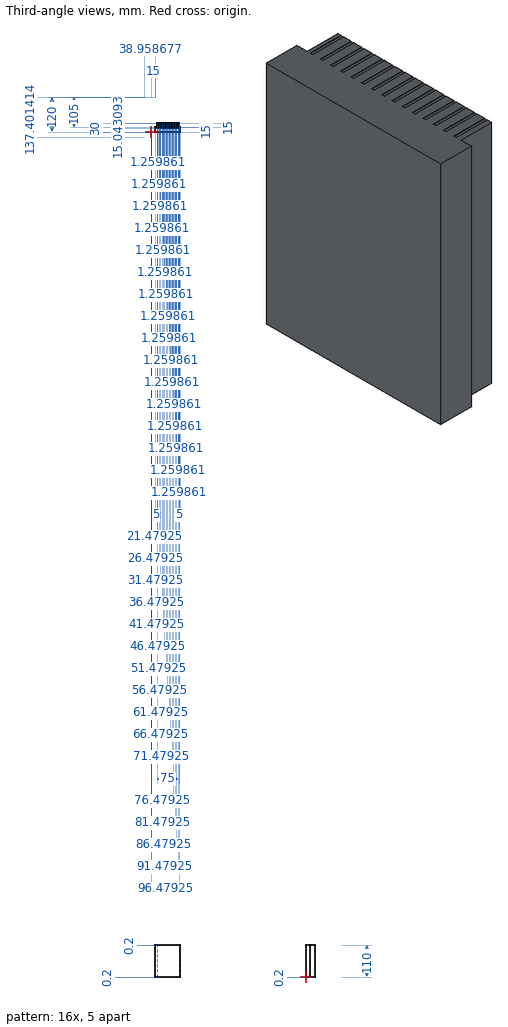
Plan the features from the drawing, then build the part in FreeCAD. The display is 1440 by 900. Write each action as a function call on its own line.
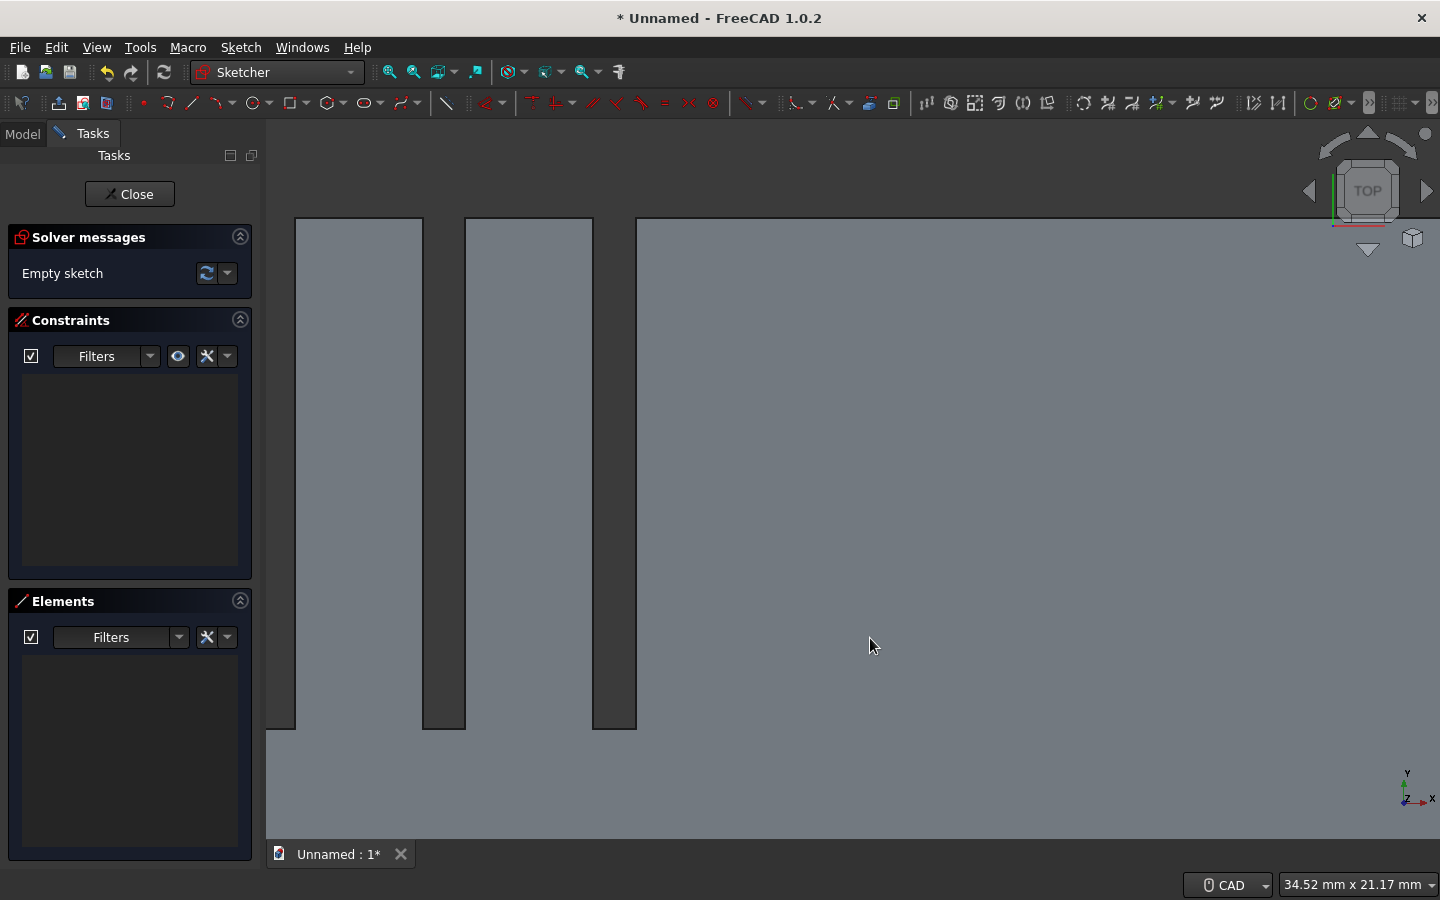
key(g)
key(r)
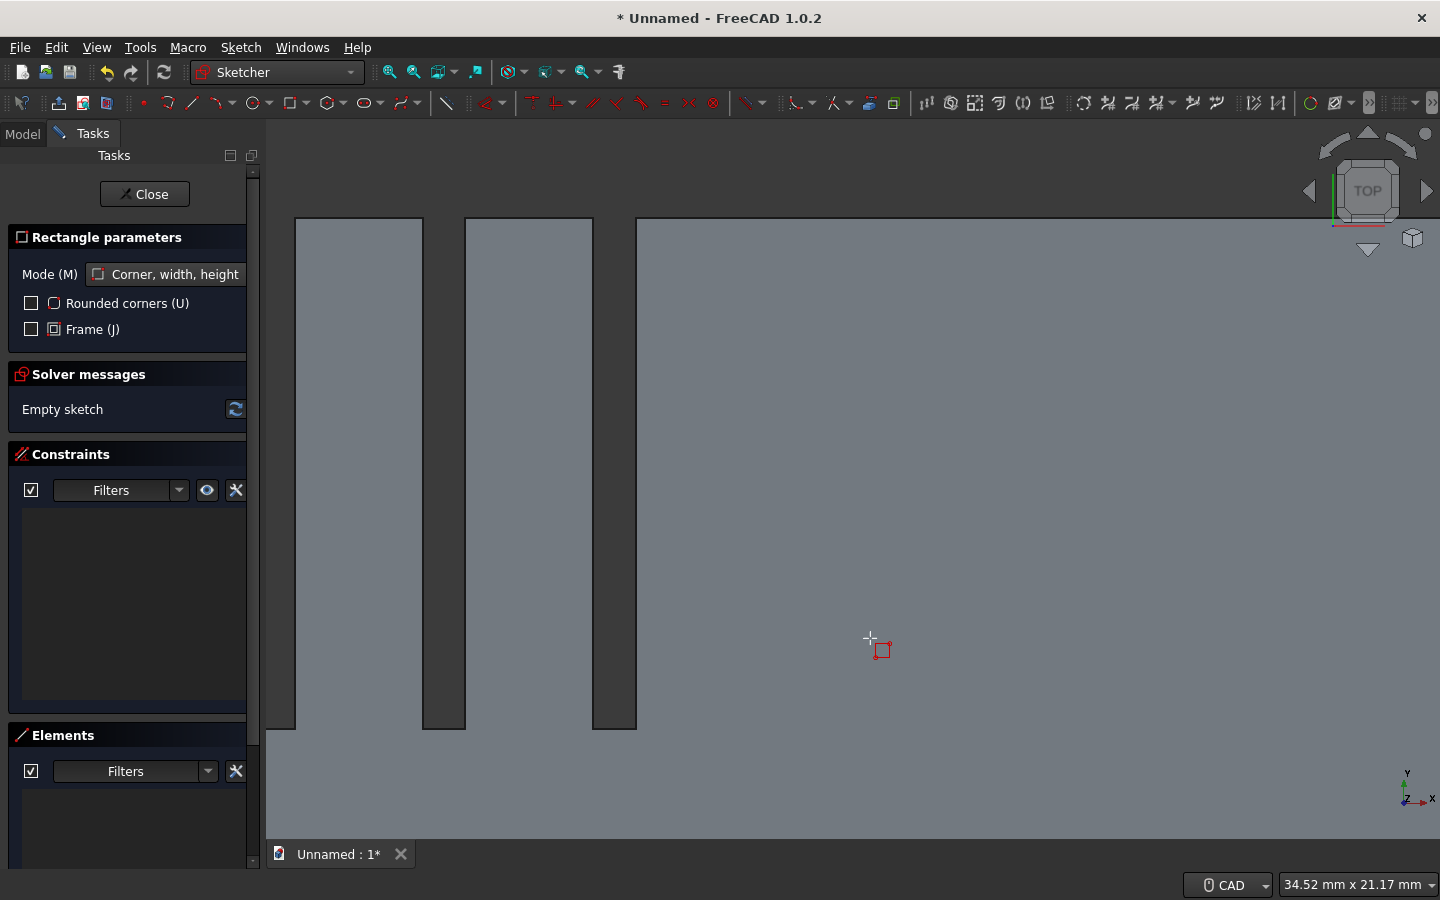
click(763, 218)
click(806, 729)
key(Escape)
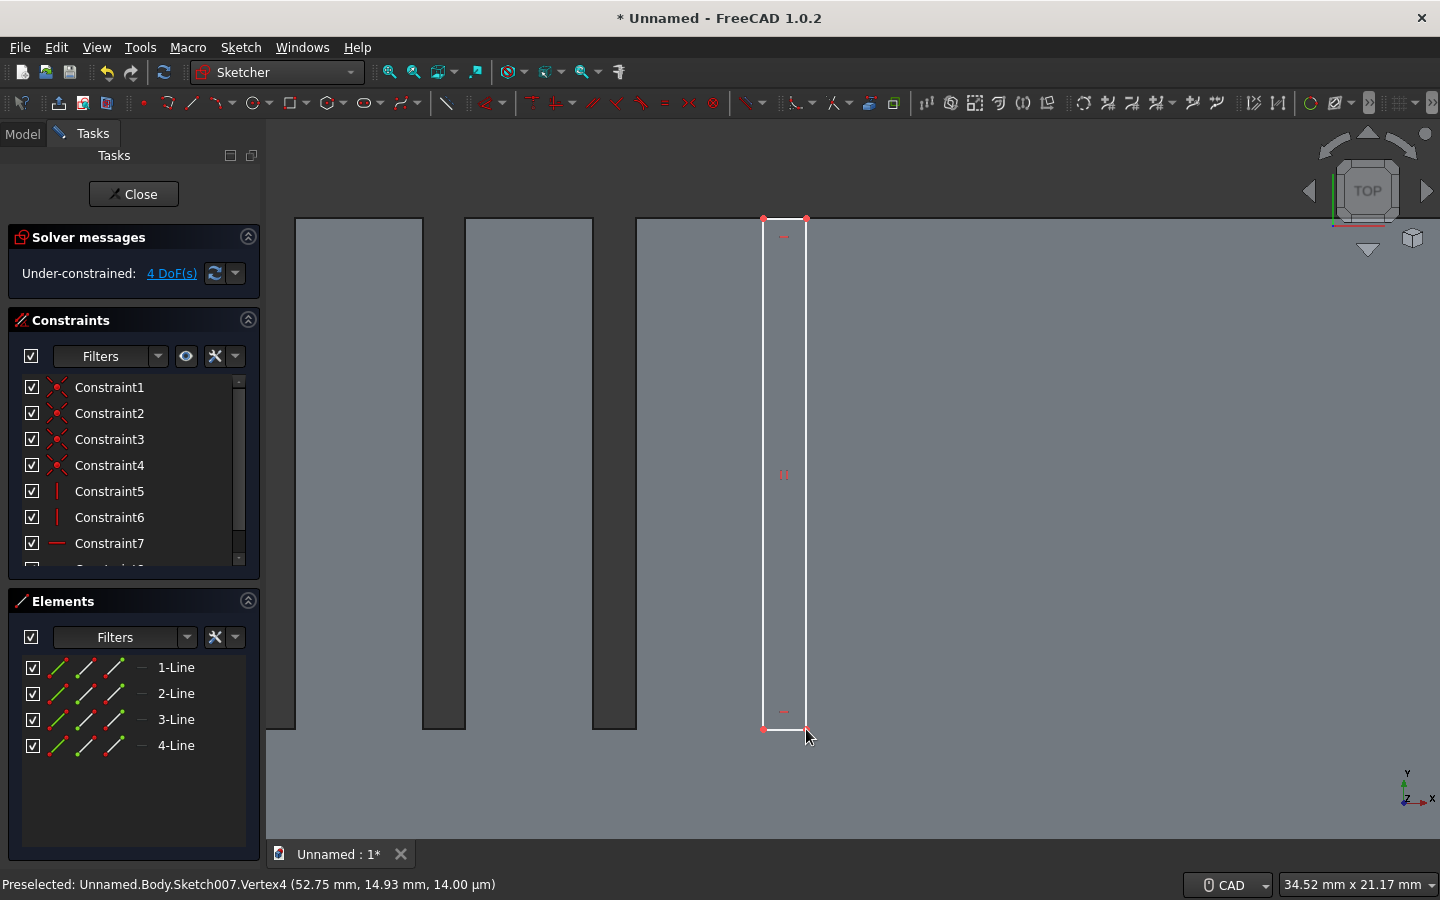
key(d)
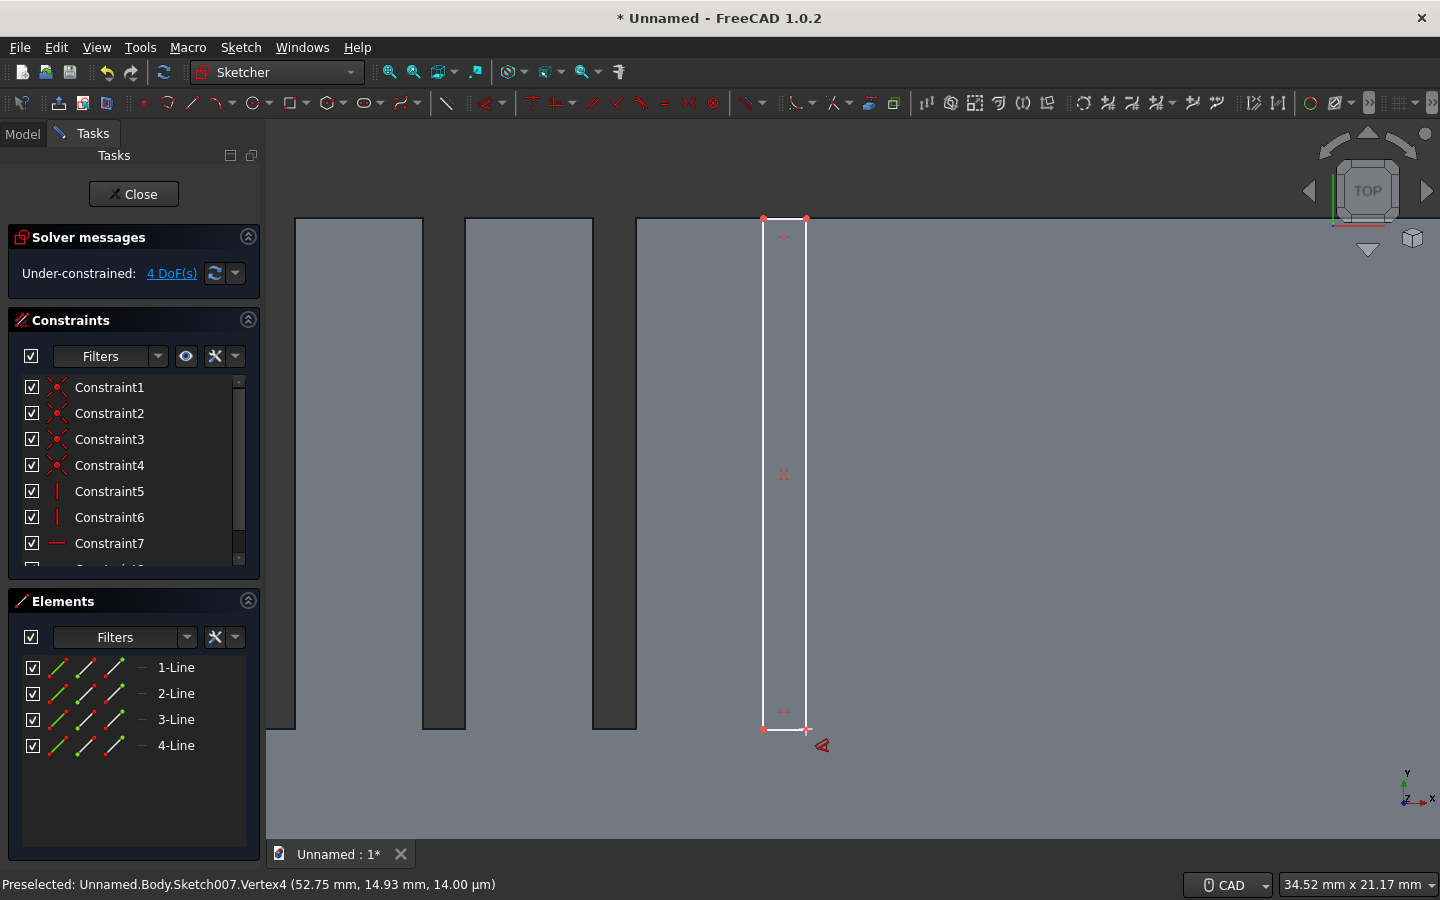
click(763, 219)
click(821, 515)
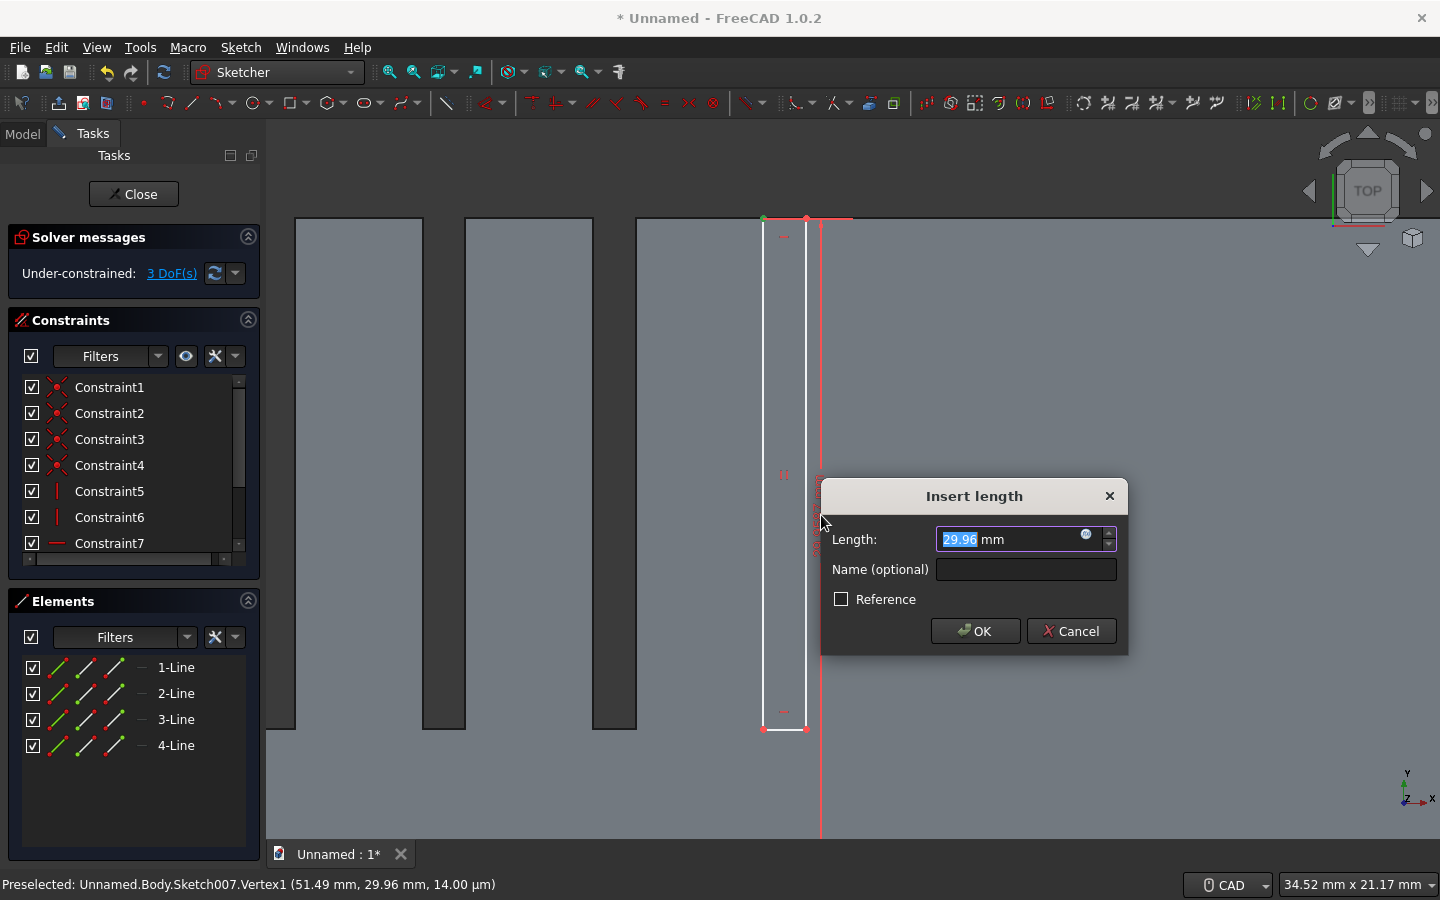
text(30)
key(Return)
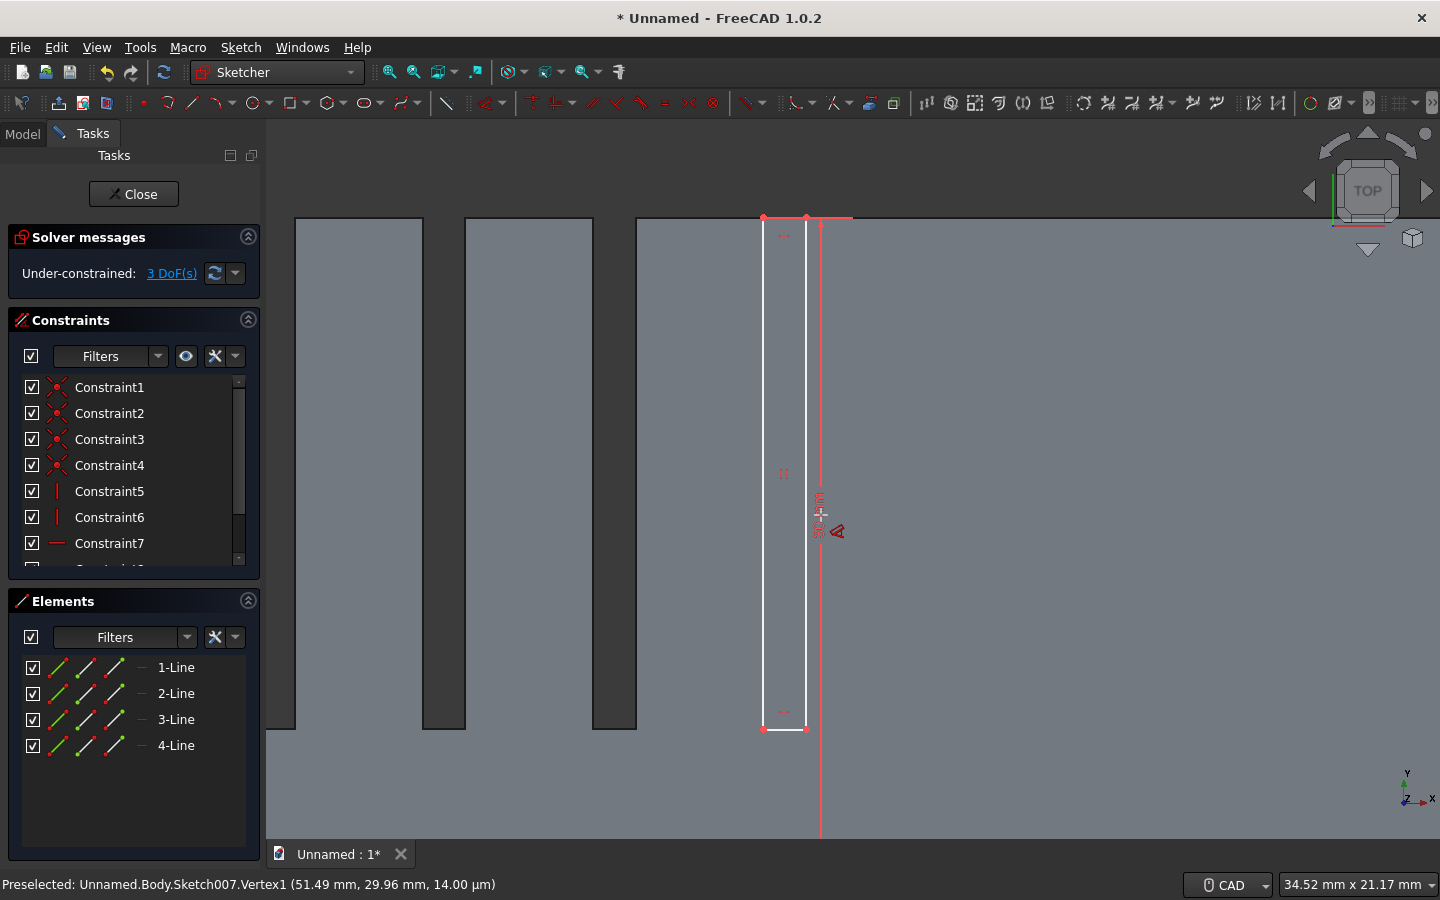
click(776, 730)
click(784, 764)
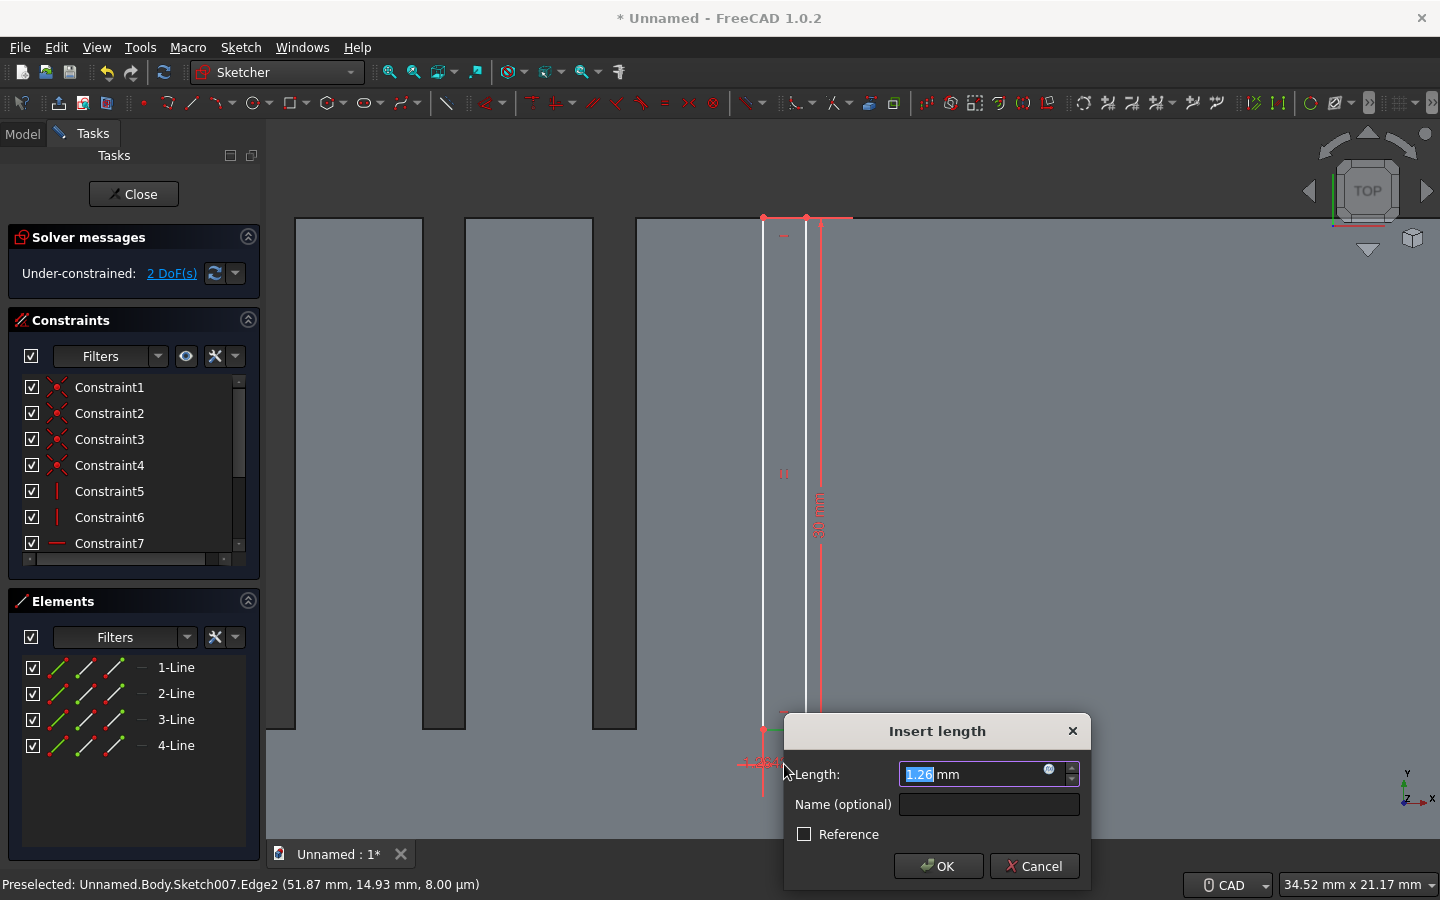
text(1.259861)
key(Return)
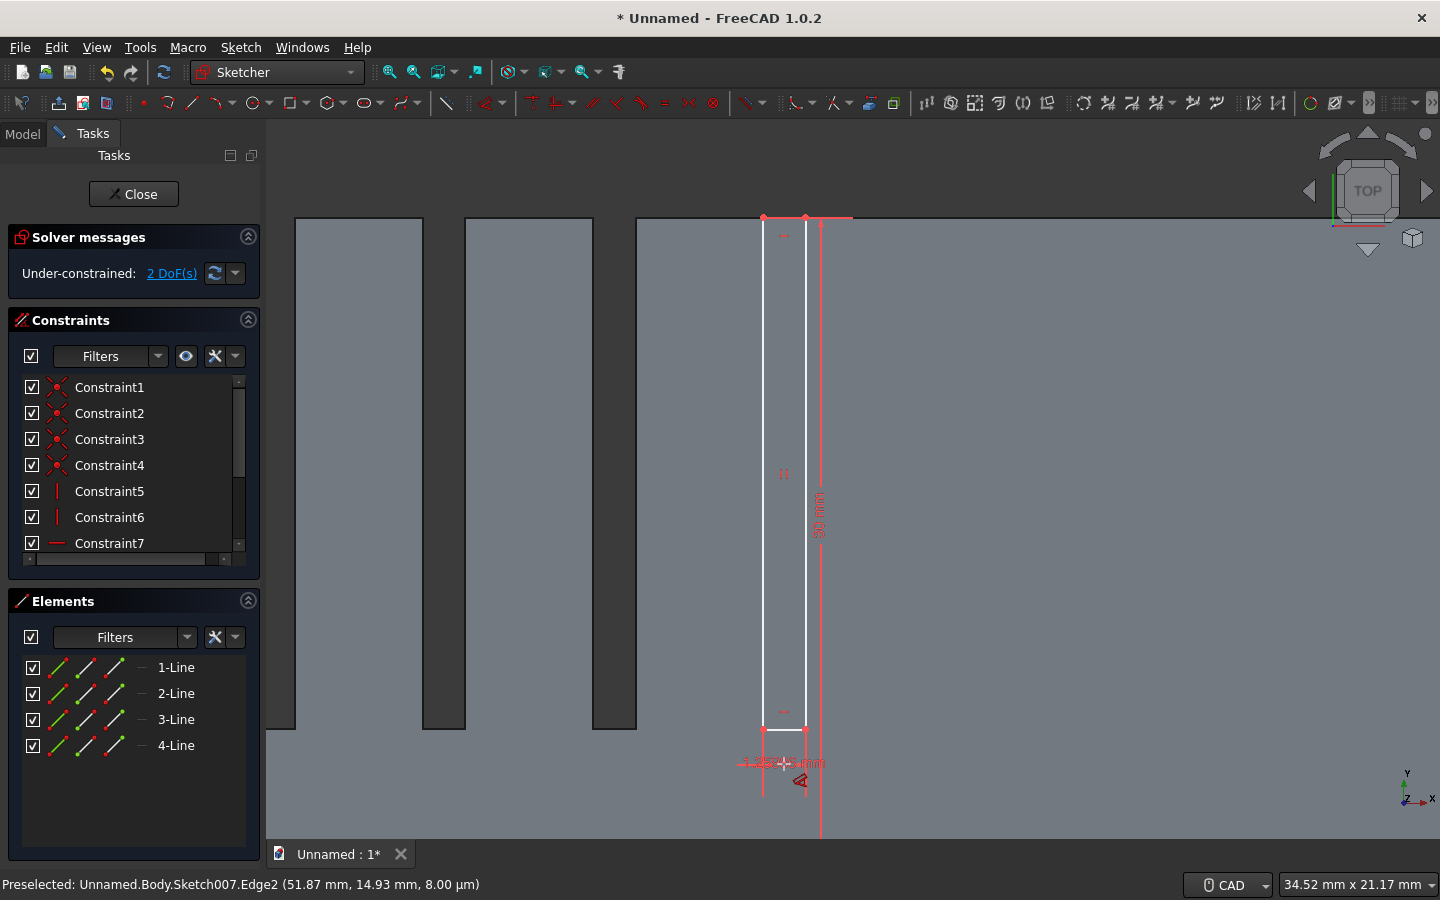
click(763, 371)
click(729, 474)